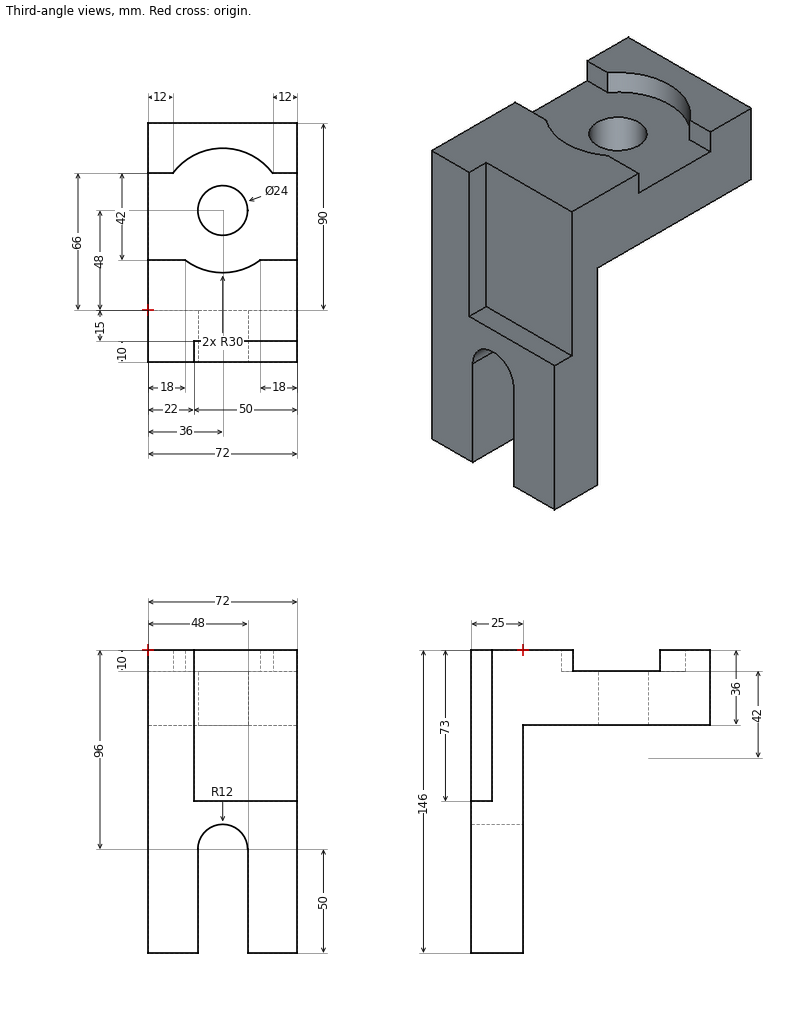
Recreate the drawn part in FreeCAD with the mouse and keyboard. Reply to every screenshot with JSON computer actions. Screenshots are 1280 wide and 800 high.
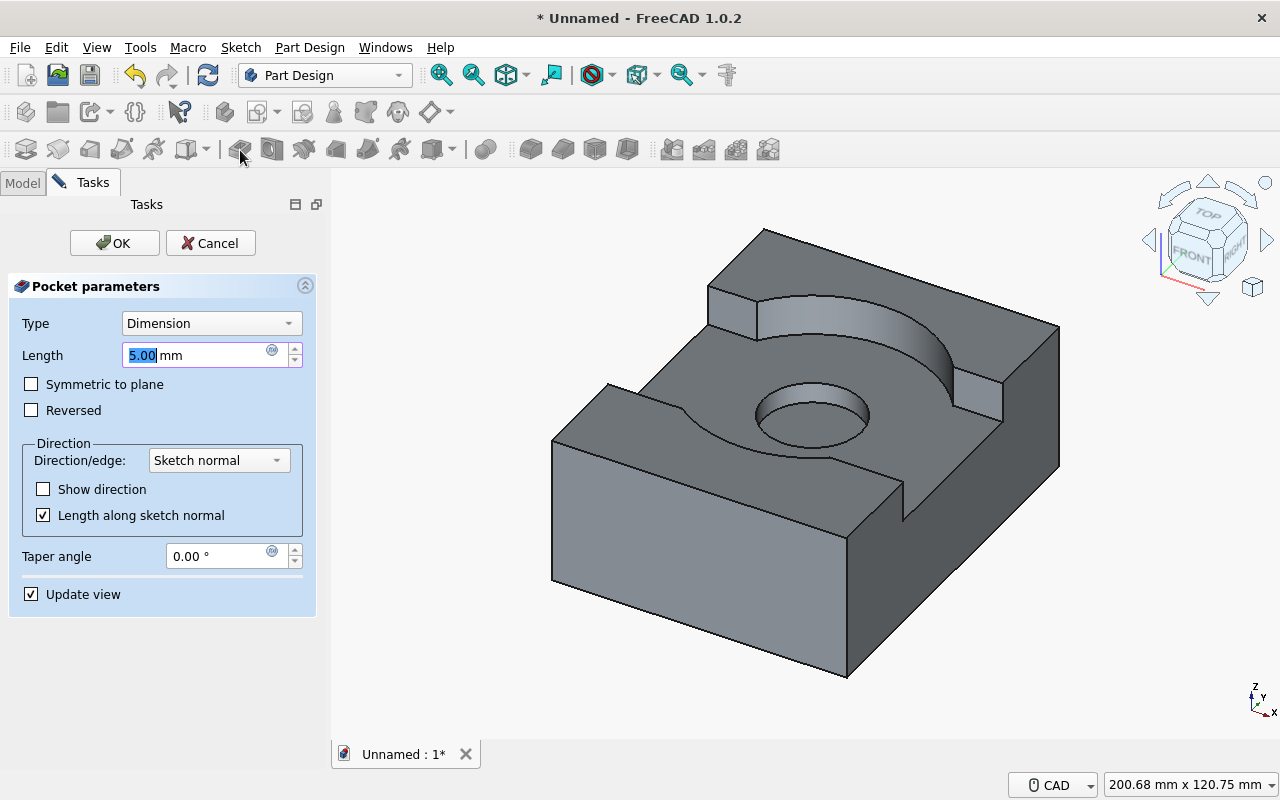
{"action": "type", "text": "42"}
{"action": "key", "text": "Tab"}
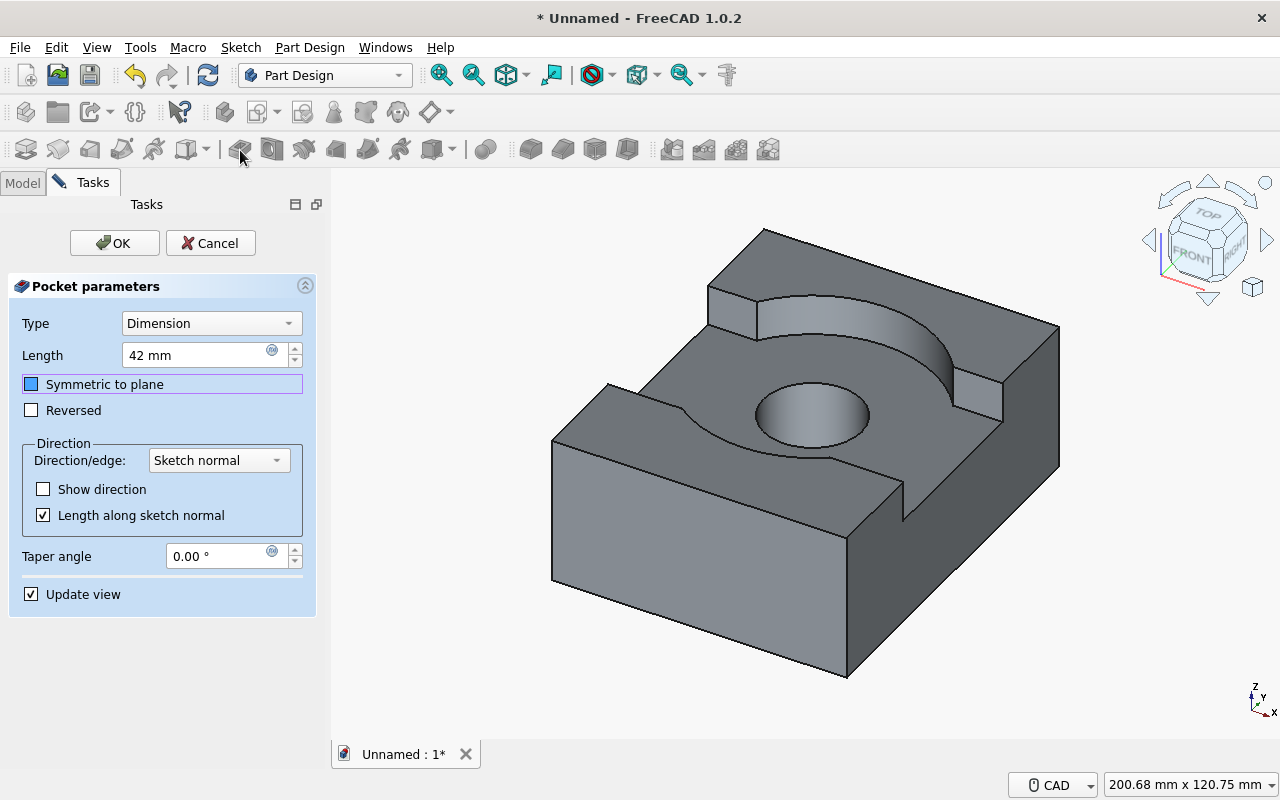
{"action": "left_click", "coordinate": [115, 243]}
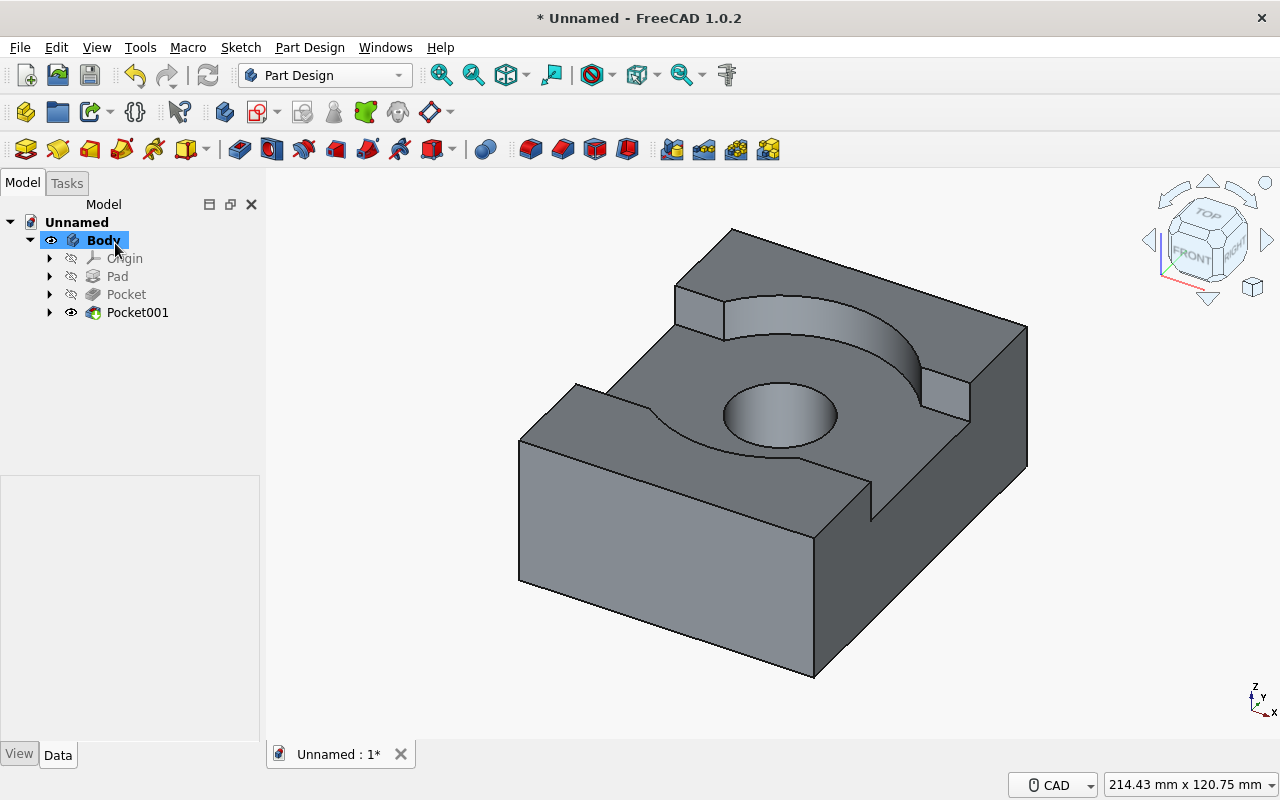
{"action": "left_click", "coordinate": [981, 461]}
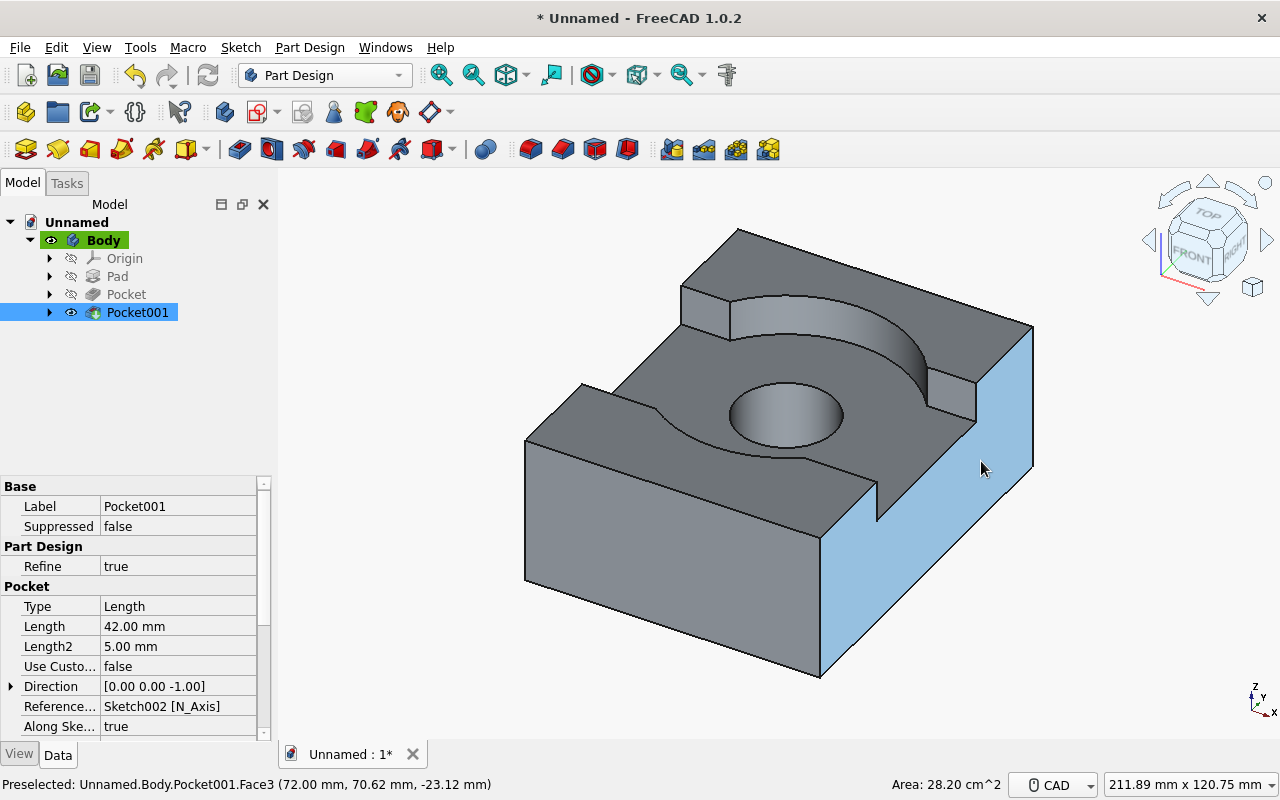
{"action": "left_click", "coordinate": [258, 112]}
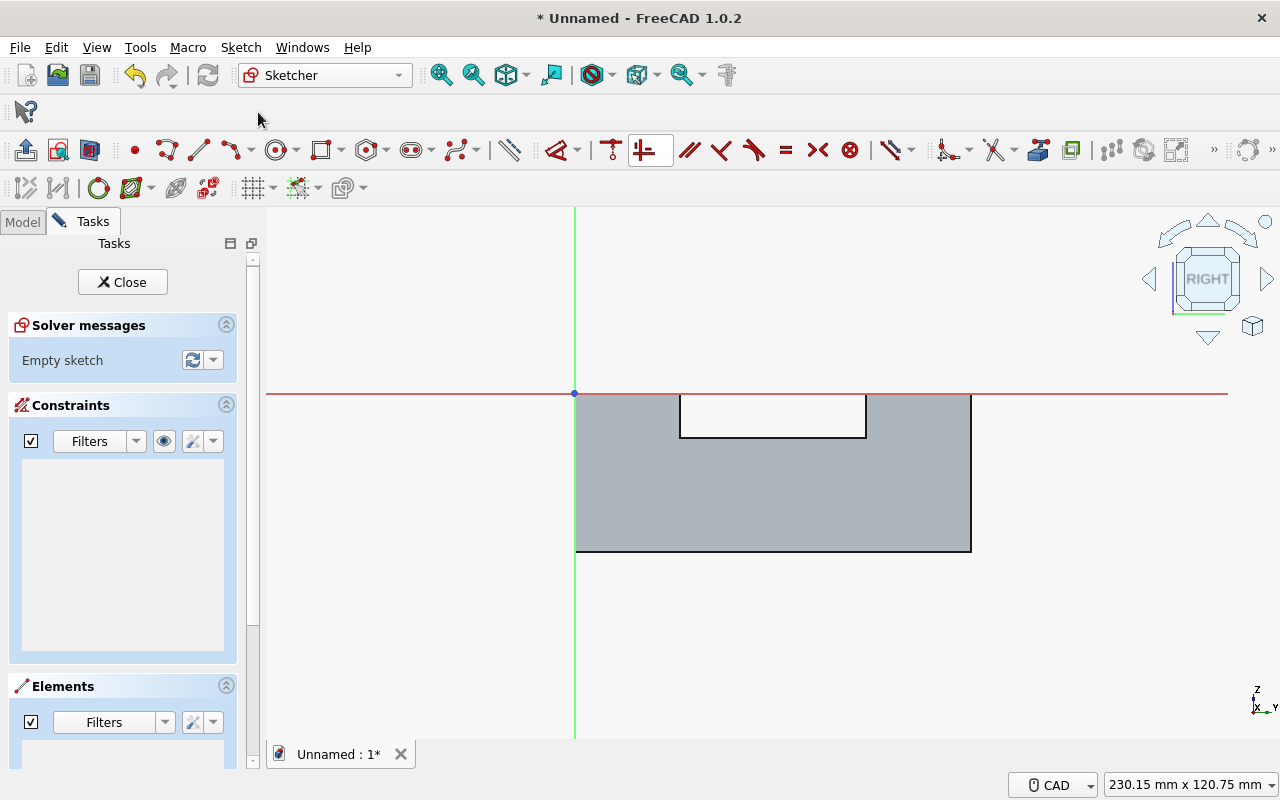
{"action": "scroll", "coordinate": [929, 235], "scroll_direction": "down", "scroll_amount": 3}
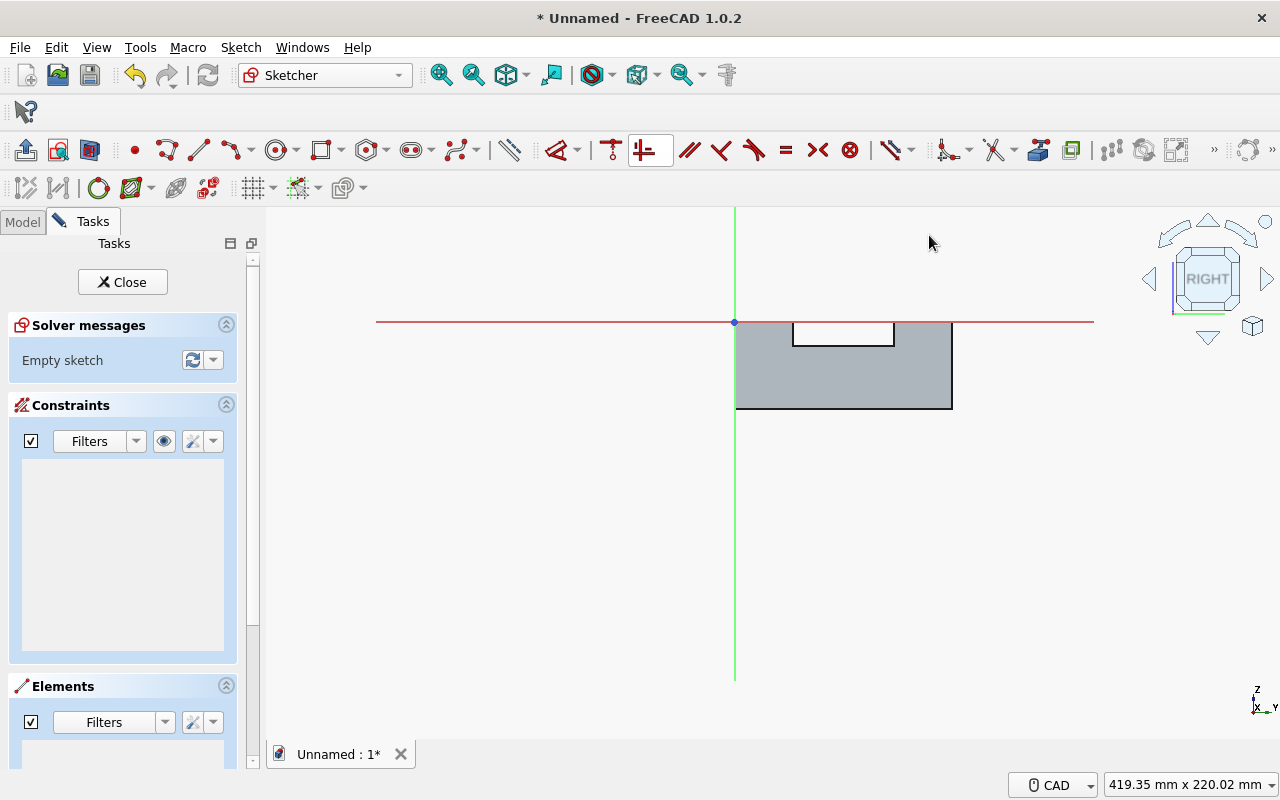
{"action": "left_click", "coordinate": [322, 150]}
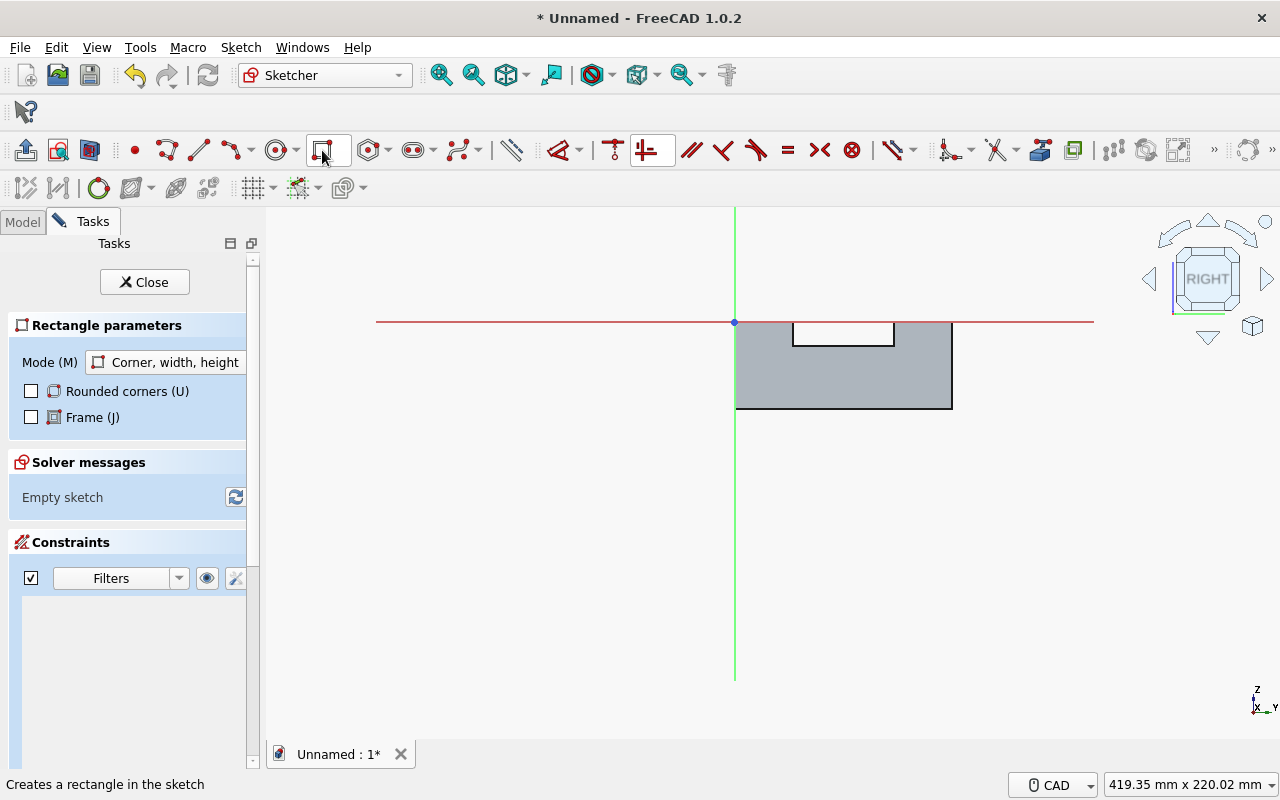
{"action": "left_click", "coordinate": [735, 322]}
{"action": "left_click", "coordinate": [674, 675]}
{"action": "key", "text": "Escape"}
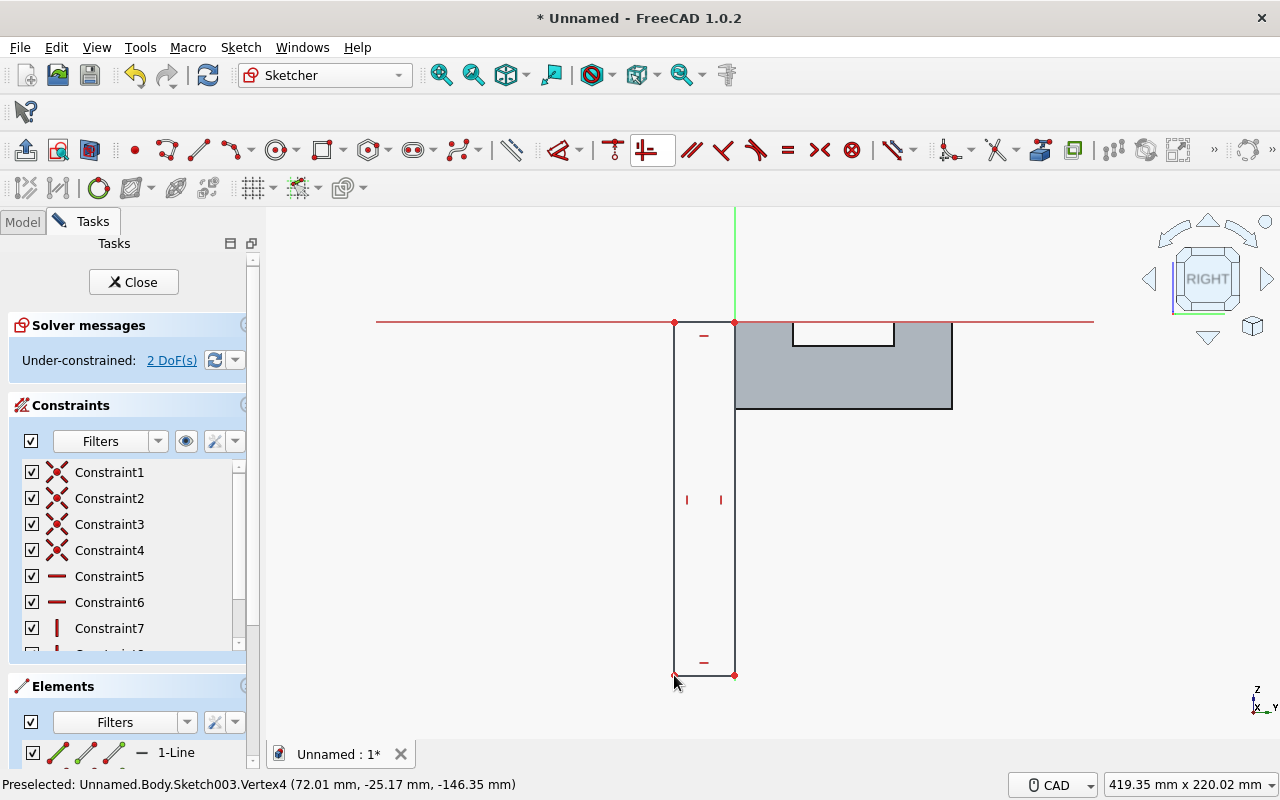
{"action": "left_click", "coordinate": [558, 150]}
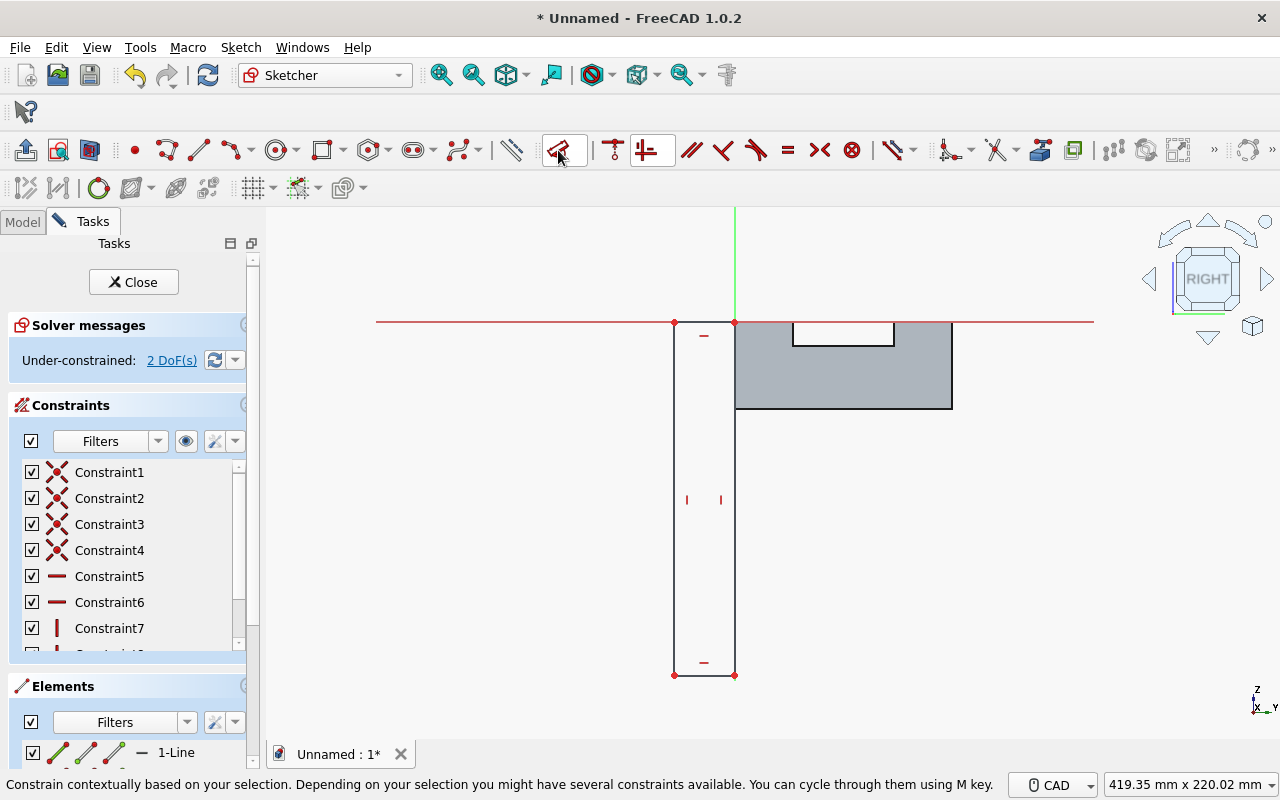
{"action": "left_click", "coordinate": [717, 322]}
{"action": "left_click", "coordinate": [704, 288]}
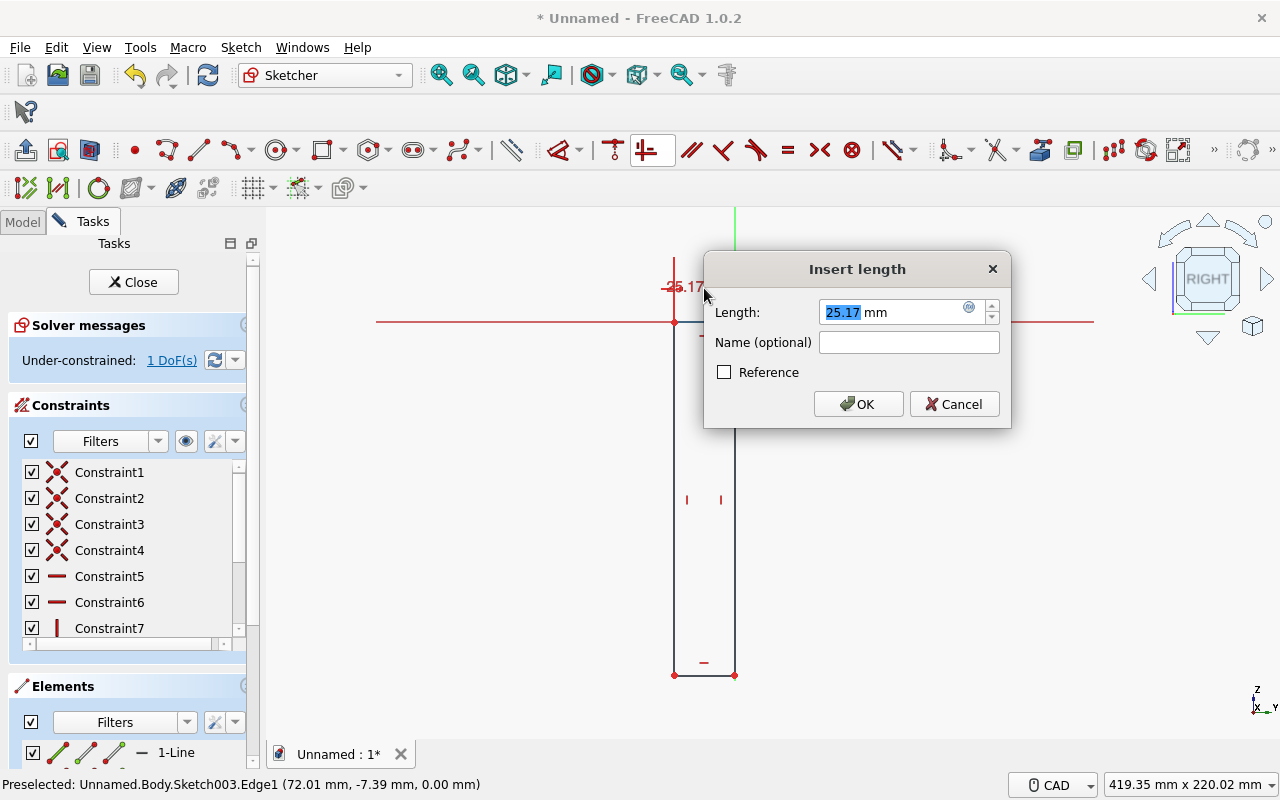
{"action": "type", "text": "25"}
{"action": "key", "text": "Return"}